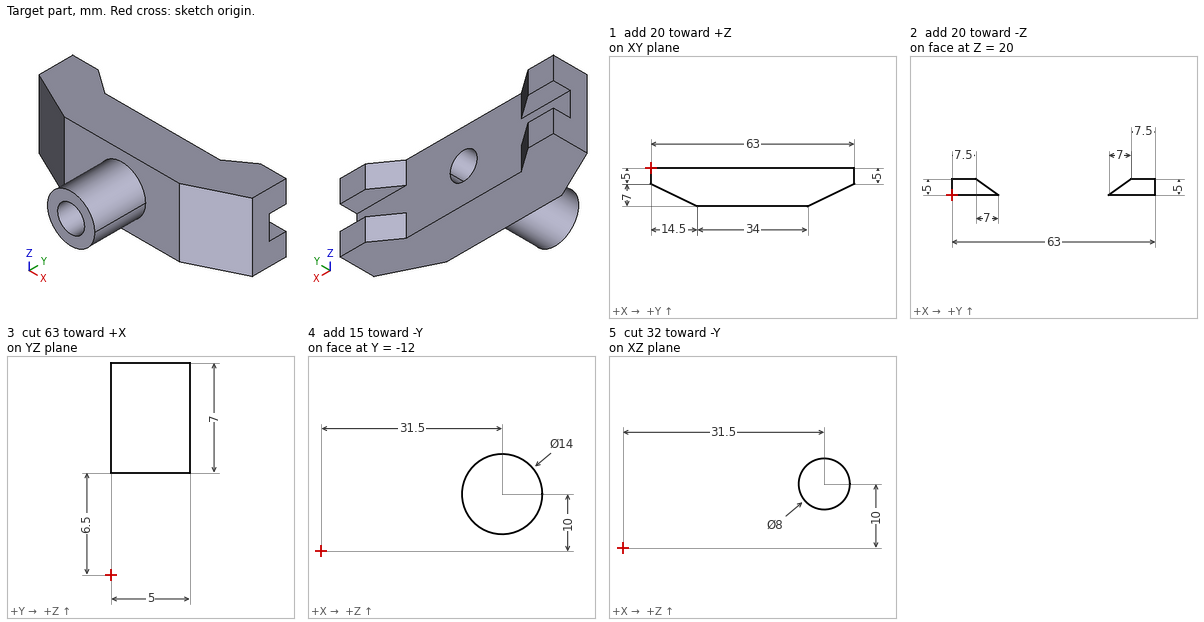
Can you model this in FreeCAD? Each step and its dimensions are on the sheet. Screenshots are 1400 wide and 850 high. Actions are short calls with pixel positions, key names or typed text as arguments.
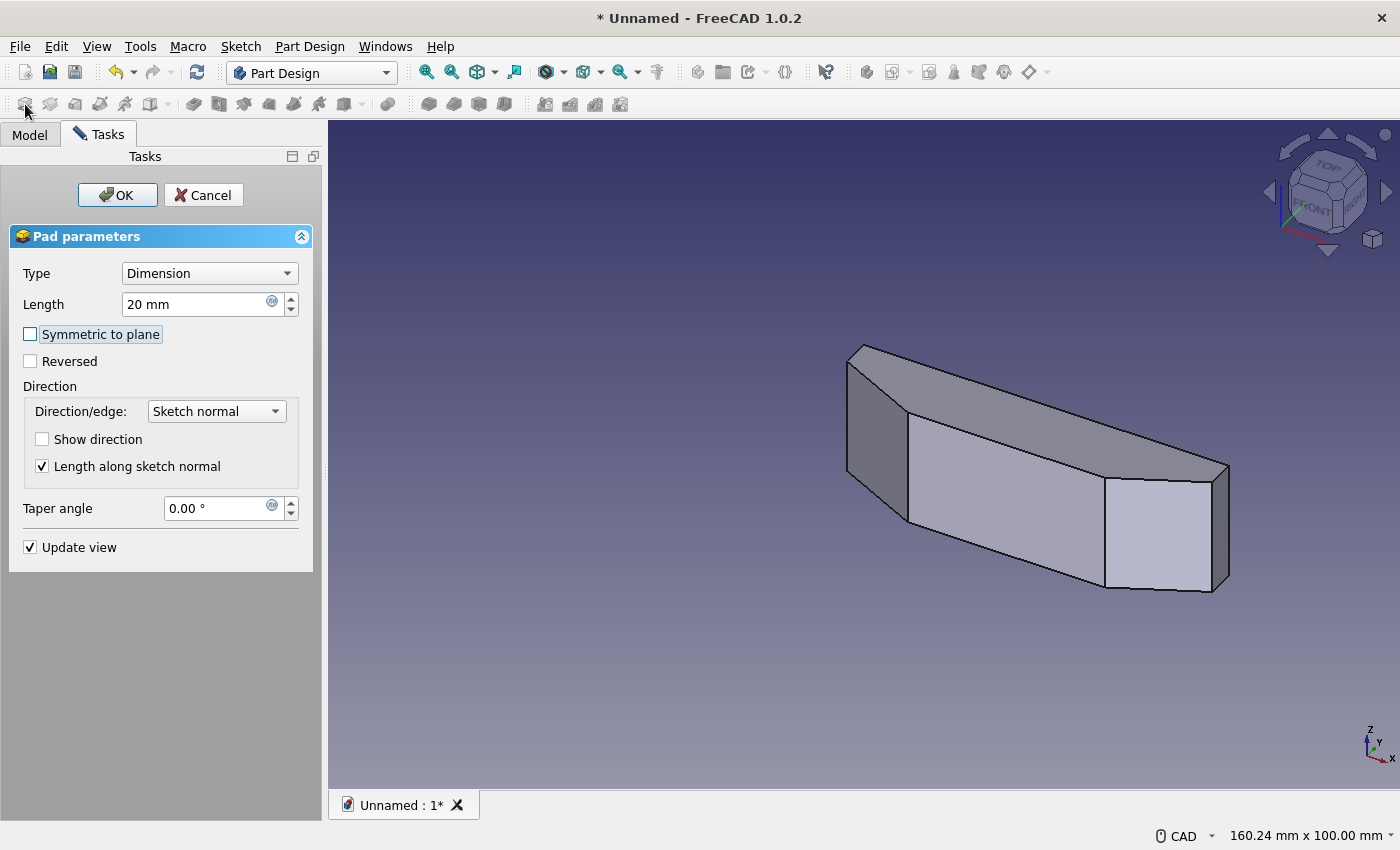
click(118, 195)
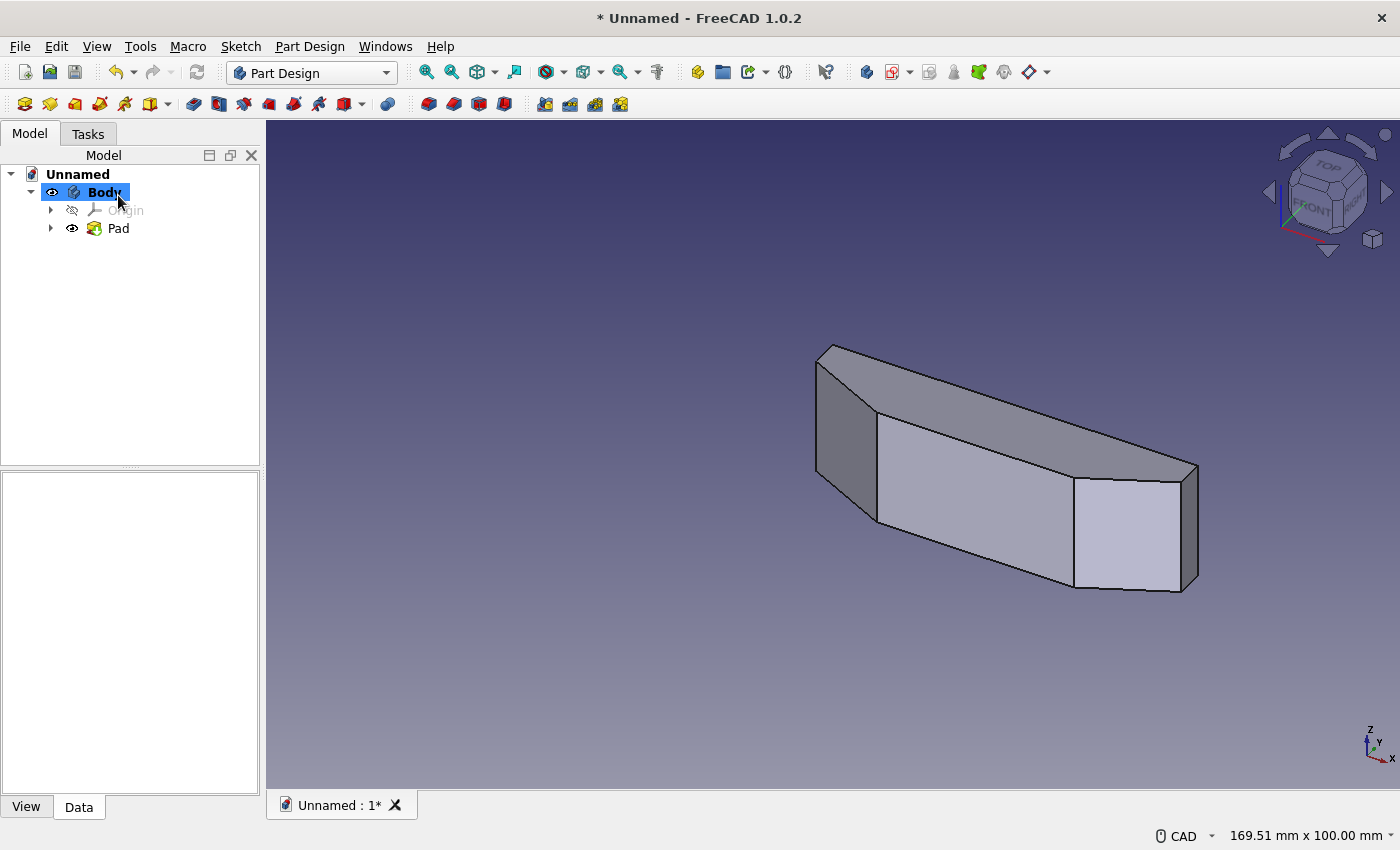
click(427, 72)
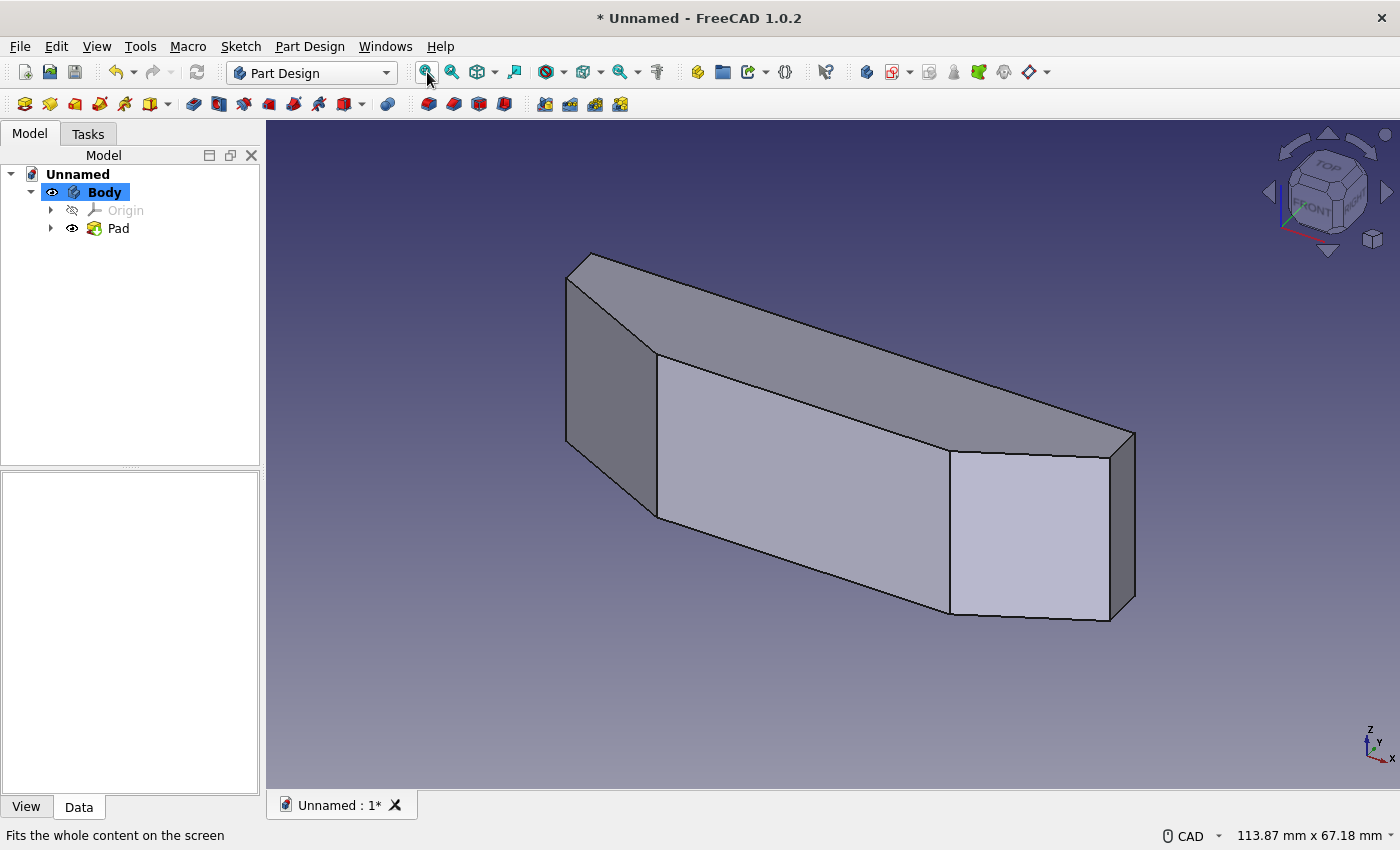
click(911, 398)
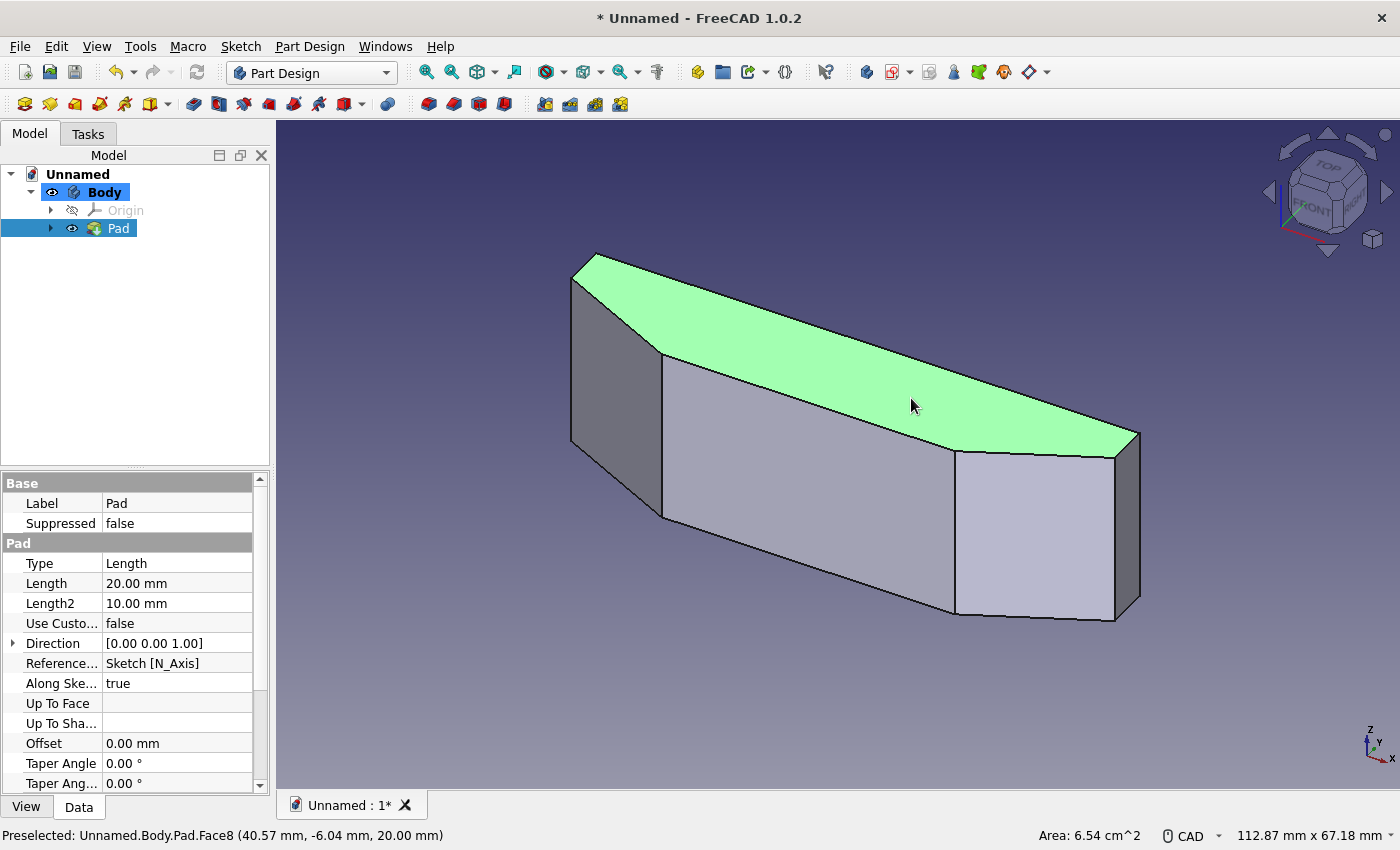
click(892, 72)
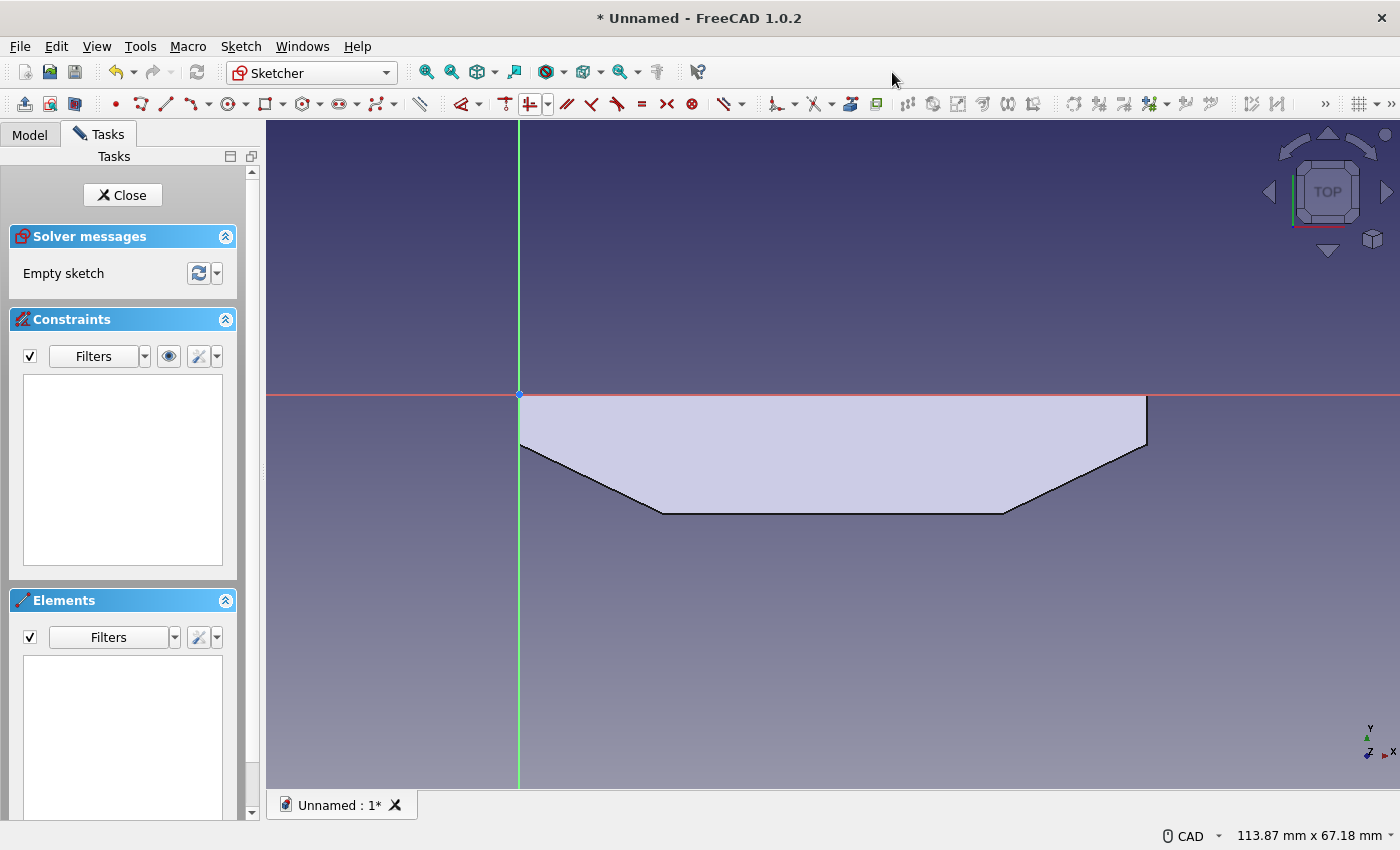
click(141, 104)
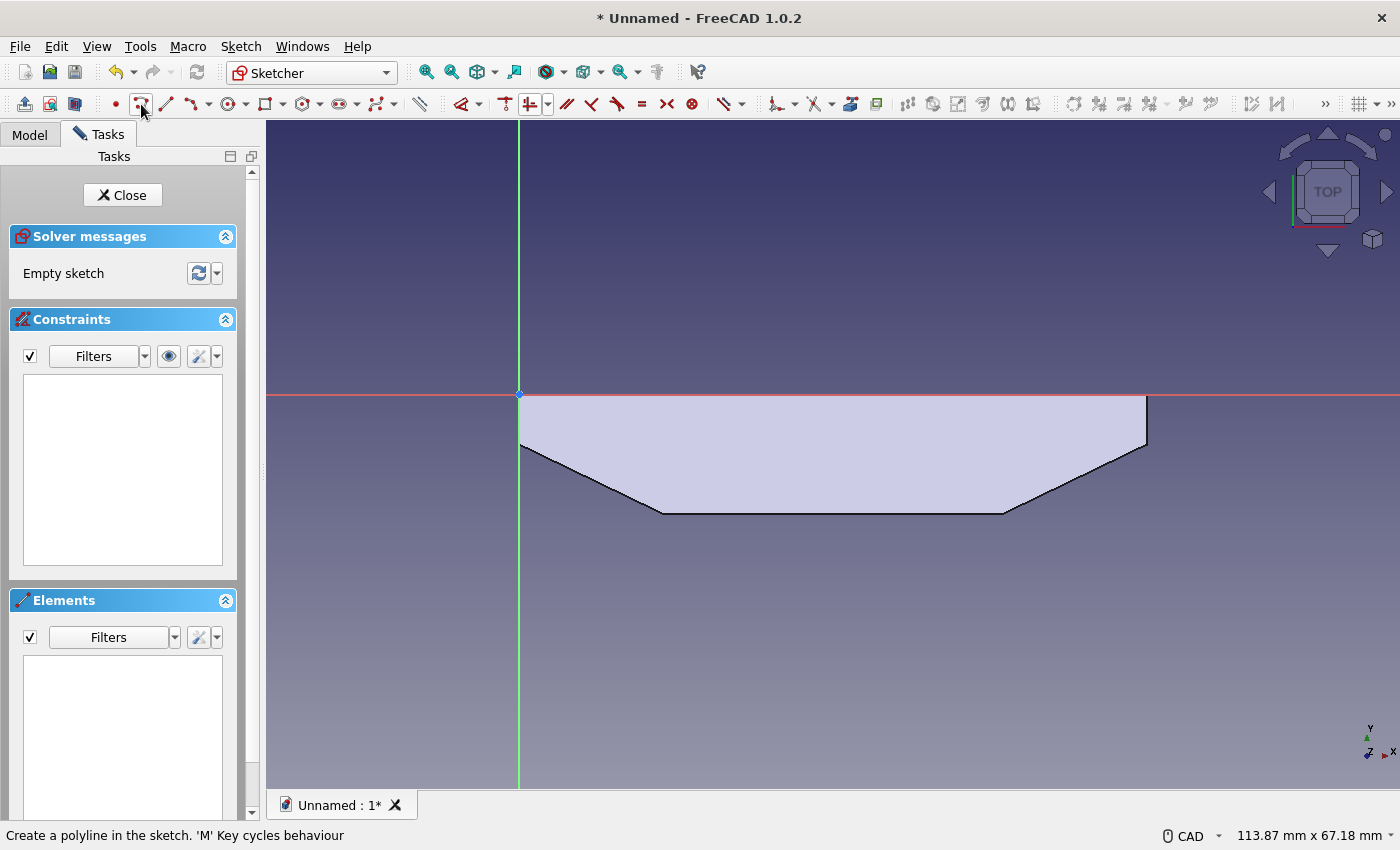
click(519, 395)
click(664, 386)
click(594, 345)
click(528, 345)
click(519, 395)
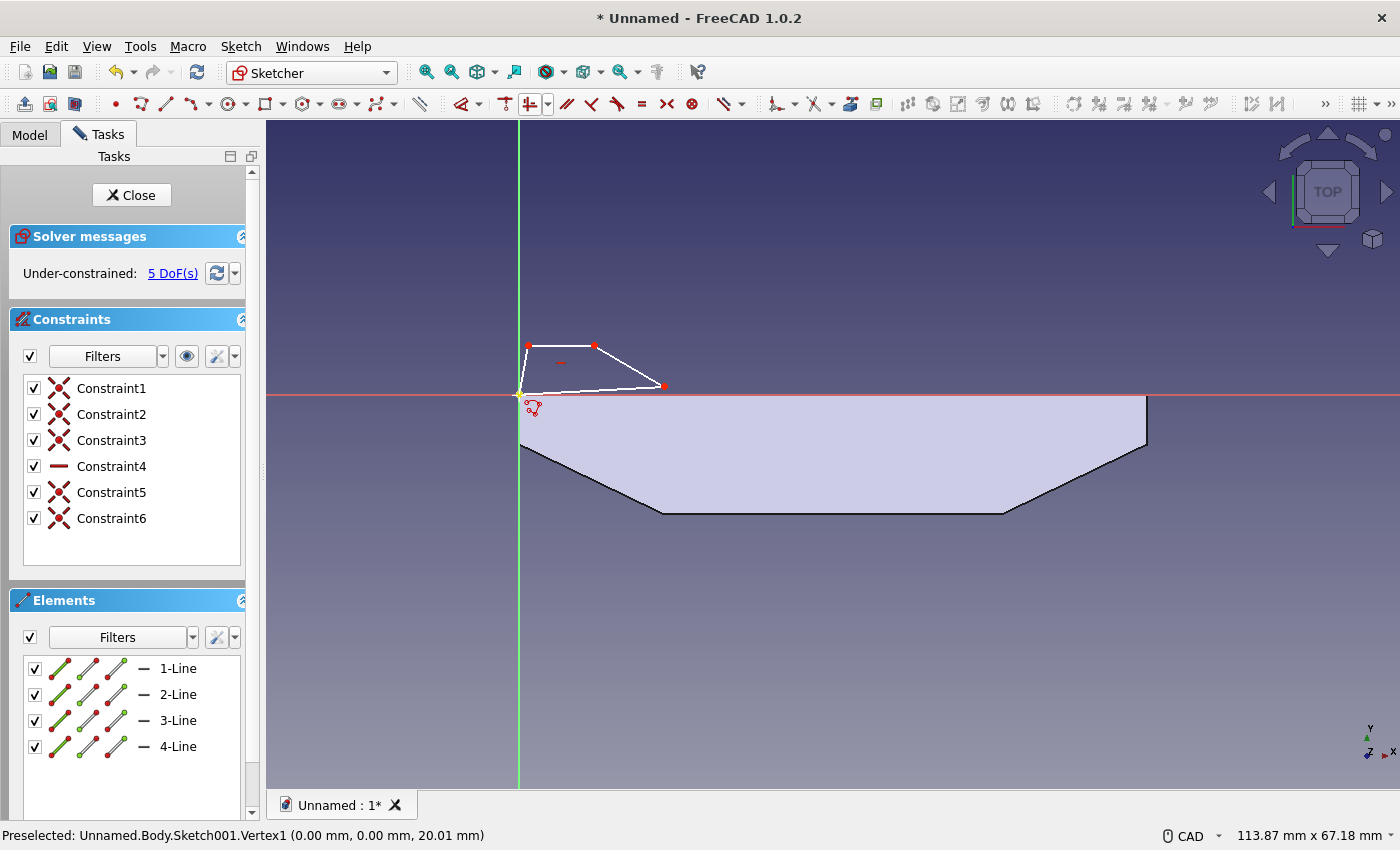
click(1002, 395)
click(1147, 386)
click(1147, 345)
click(1072, 345)
click(1002, 395)
key(Escape)
key(Escape)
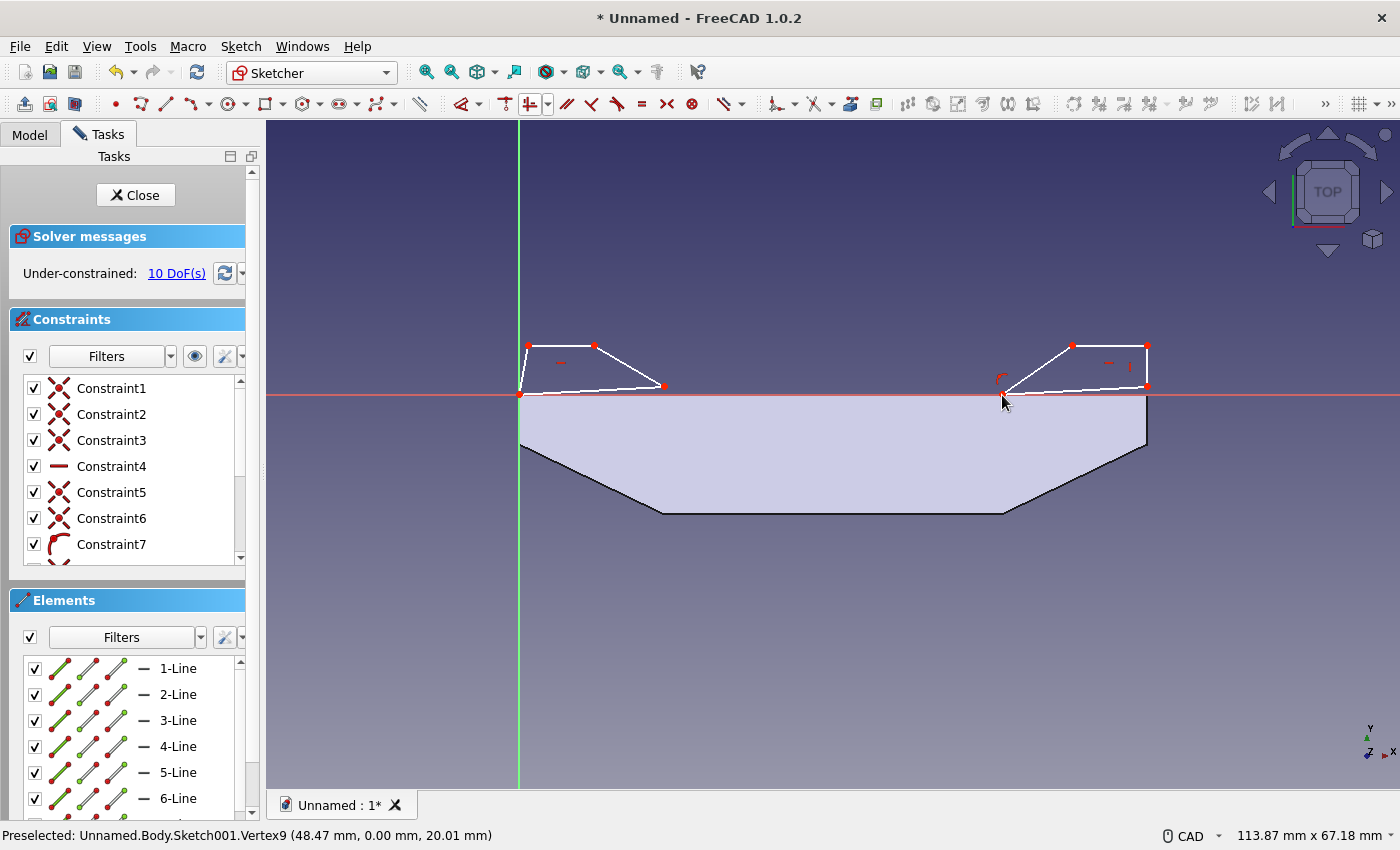
click(563, 392)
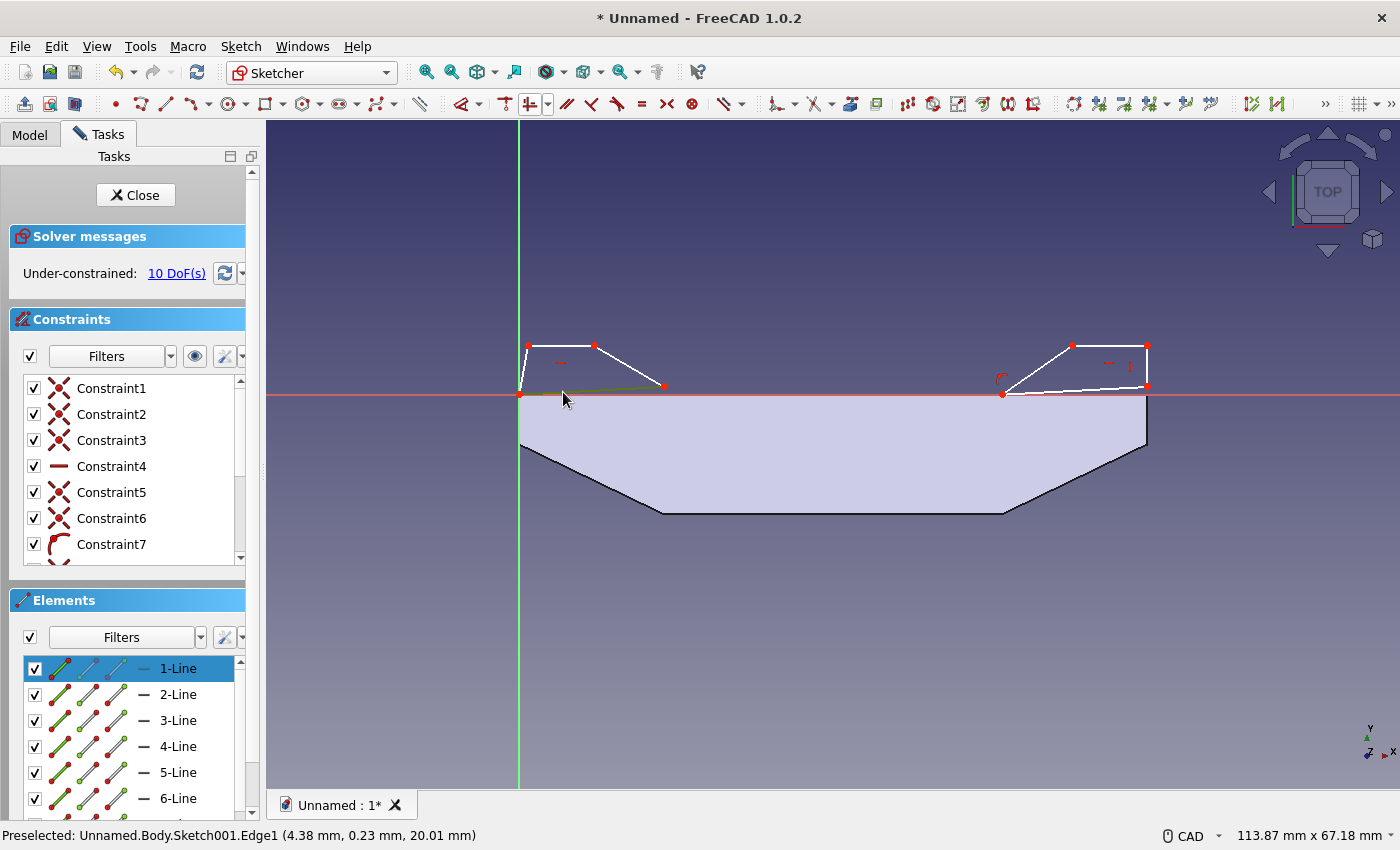
click(548, 104)